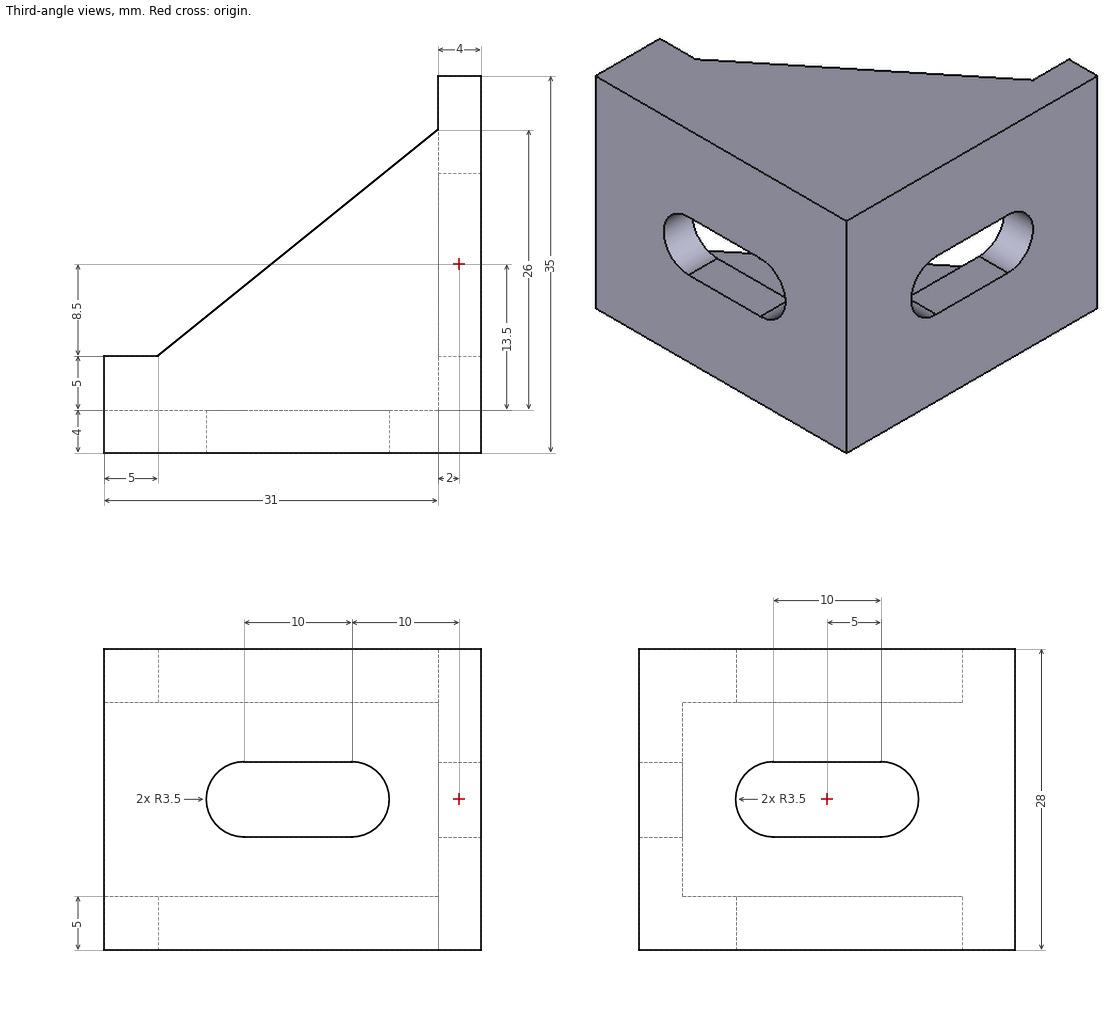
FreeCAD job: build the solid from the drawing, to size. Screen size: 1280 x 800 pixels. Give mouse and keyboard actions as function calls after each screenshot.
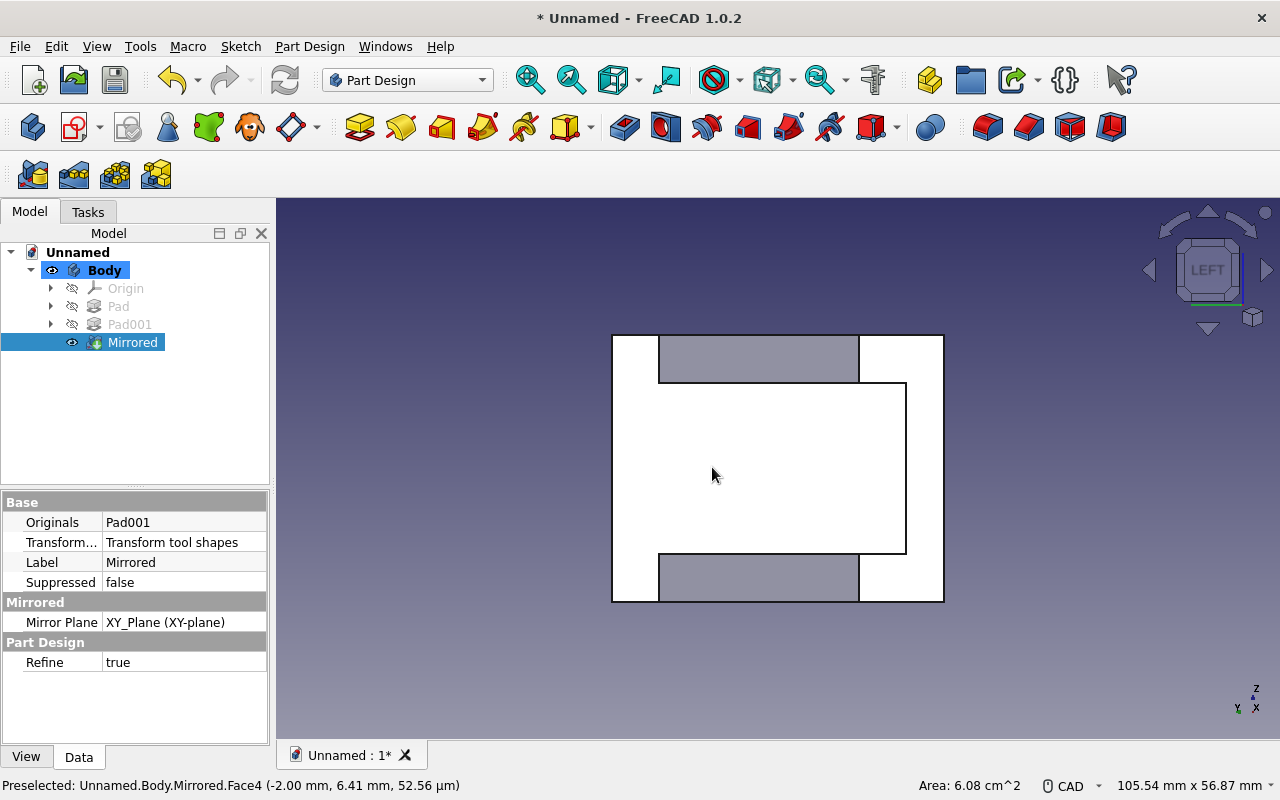
click(74, 128)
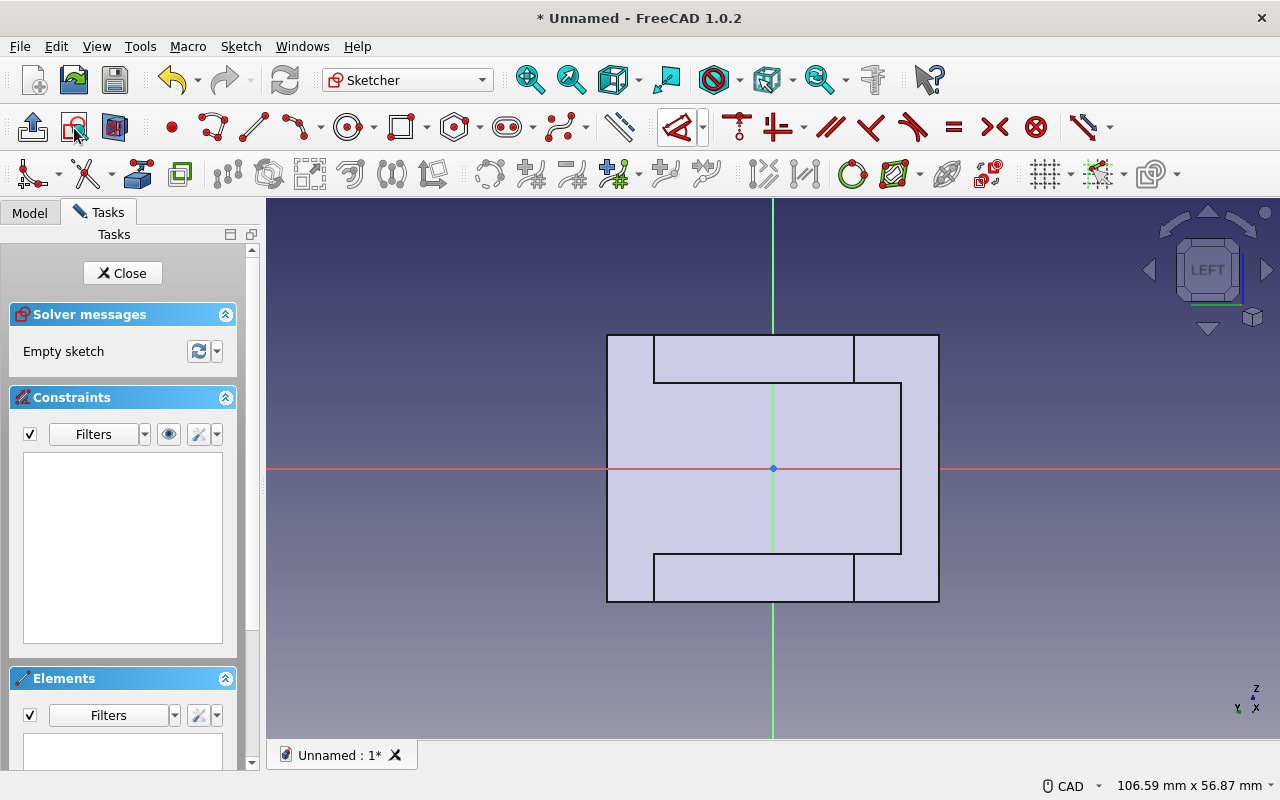
scroll(803, 468, up, 6)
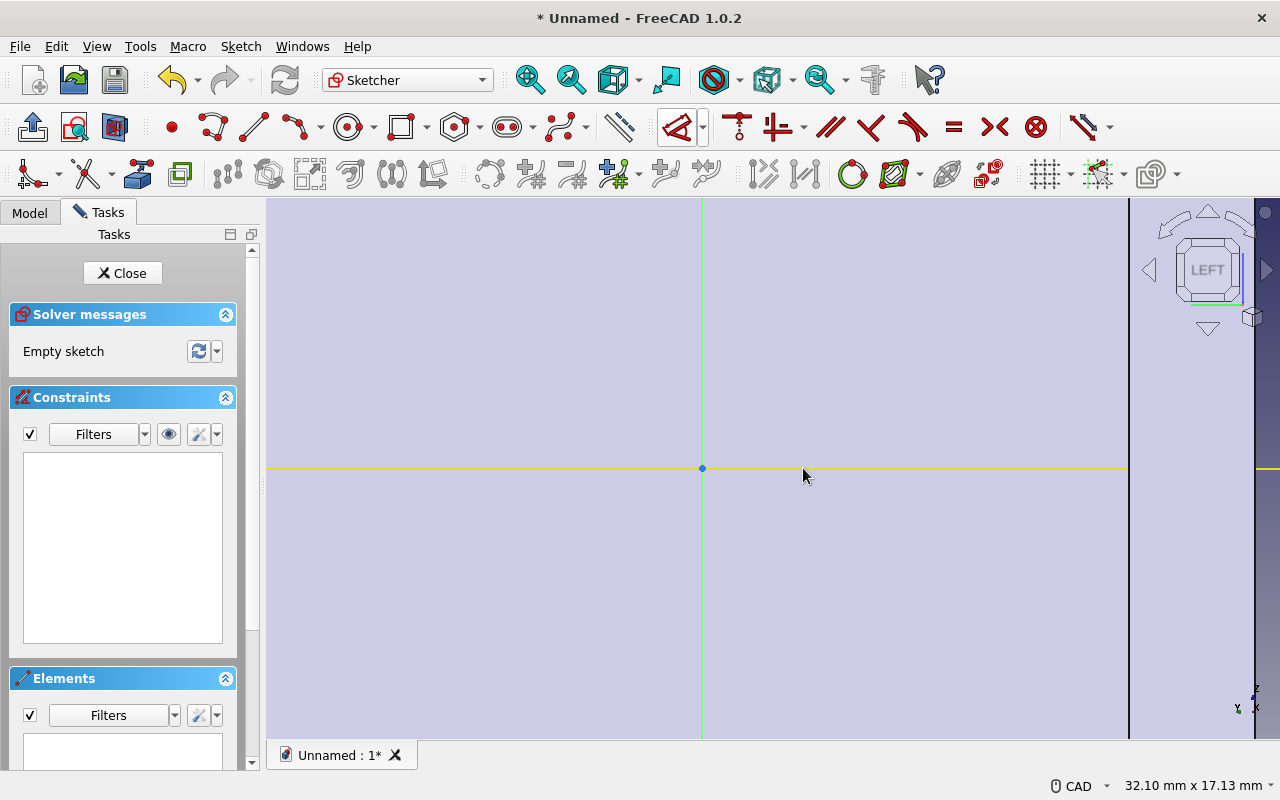
click(506, 128)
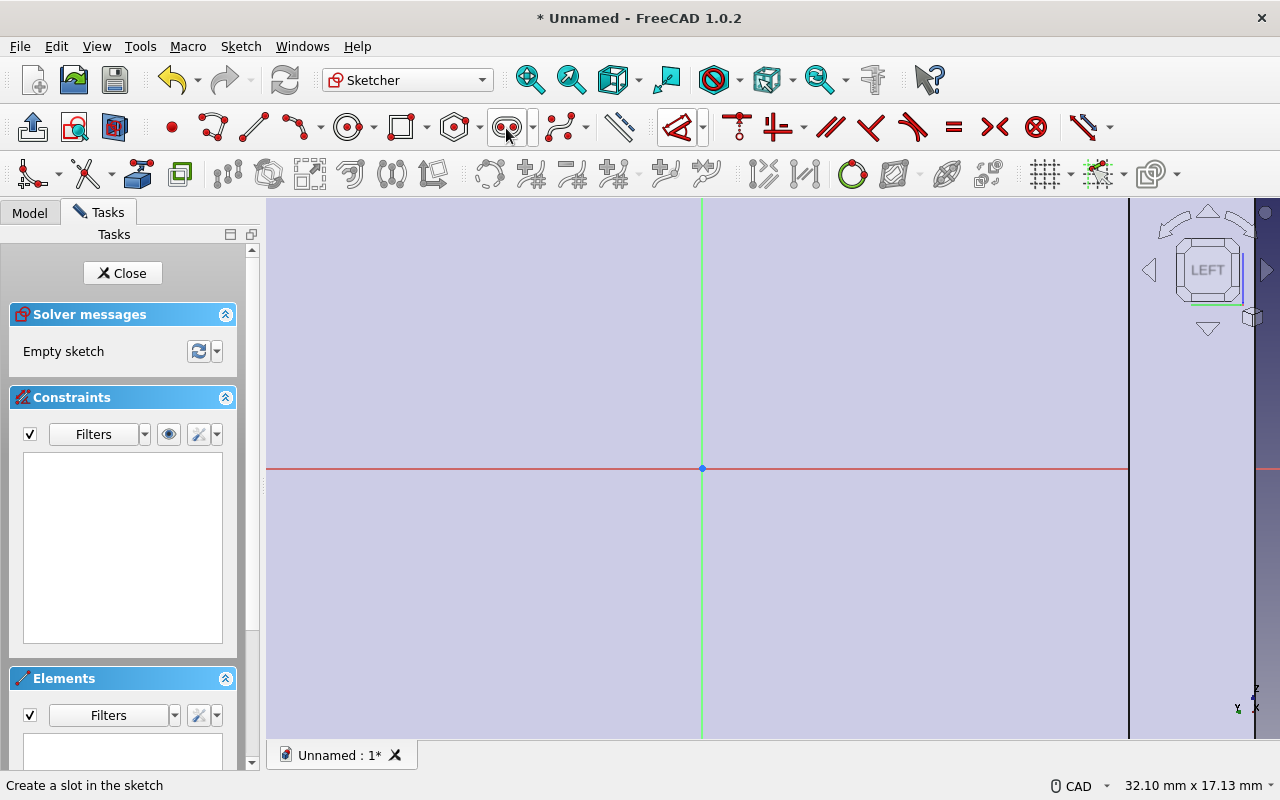
click(544, 468)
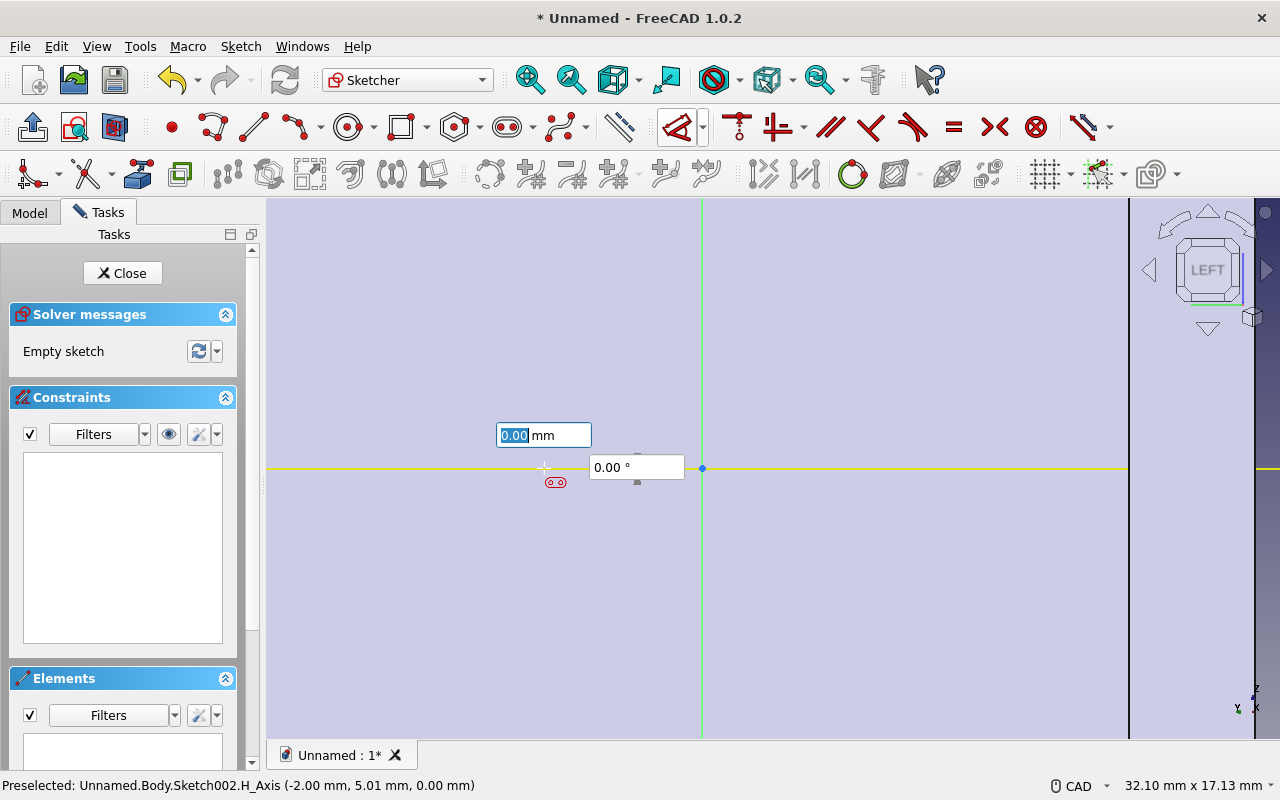
click(860, 460)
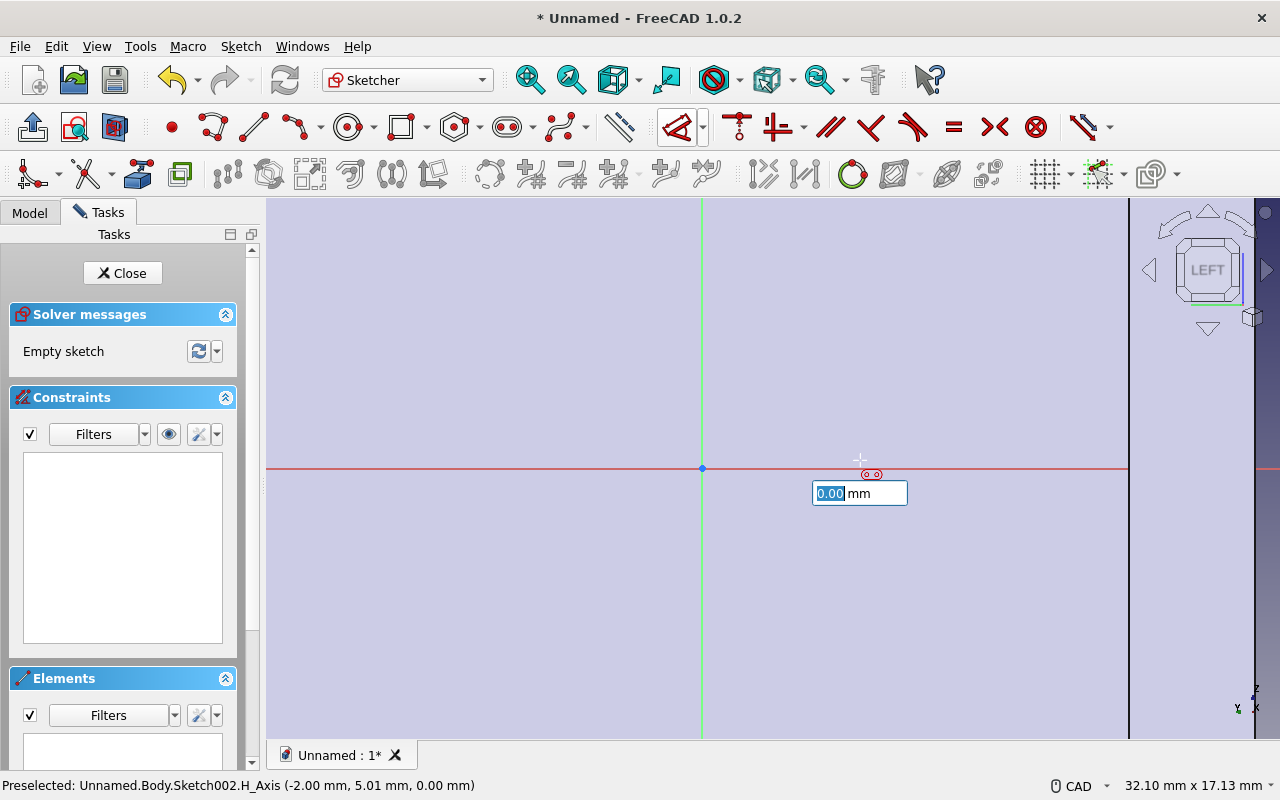
click(655, 579)
key(Escape)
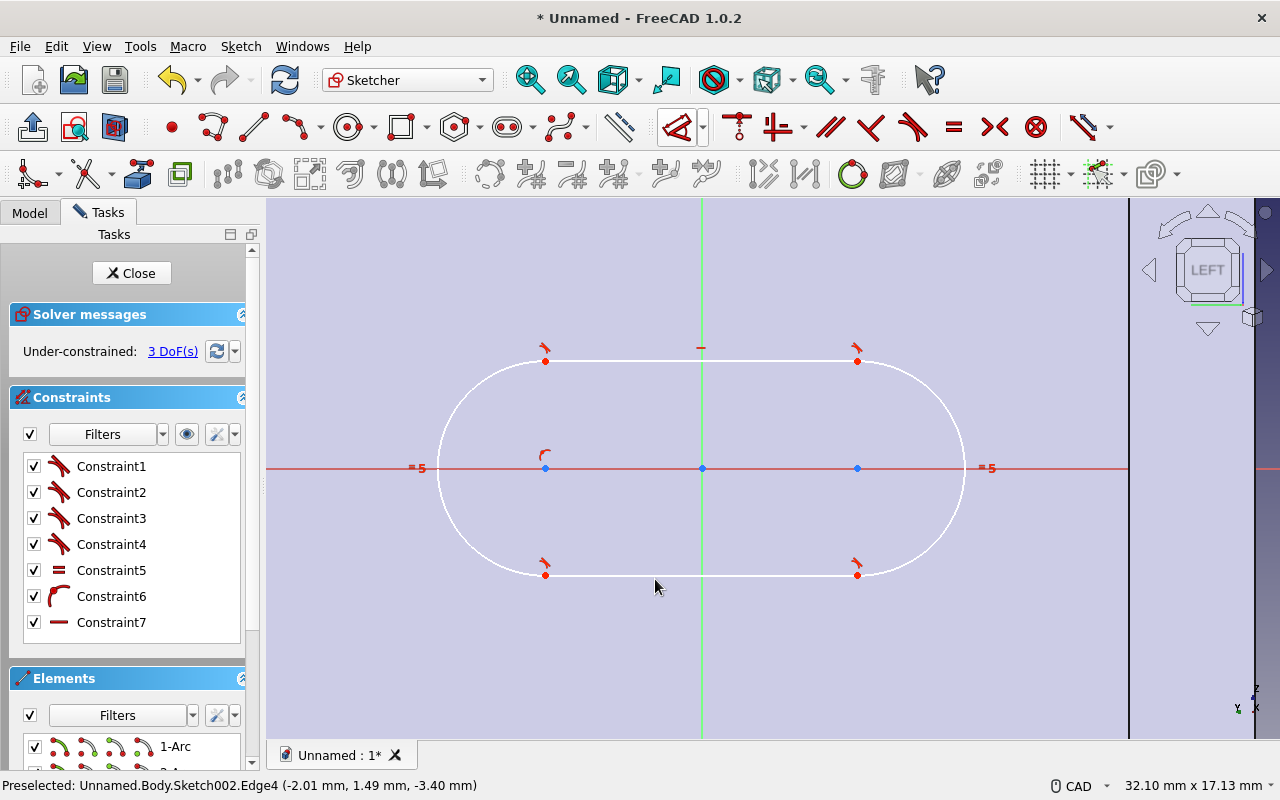
click(458, 405)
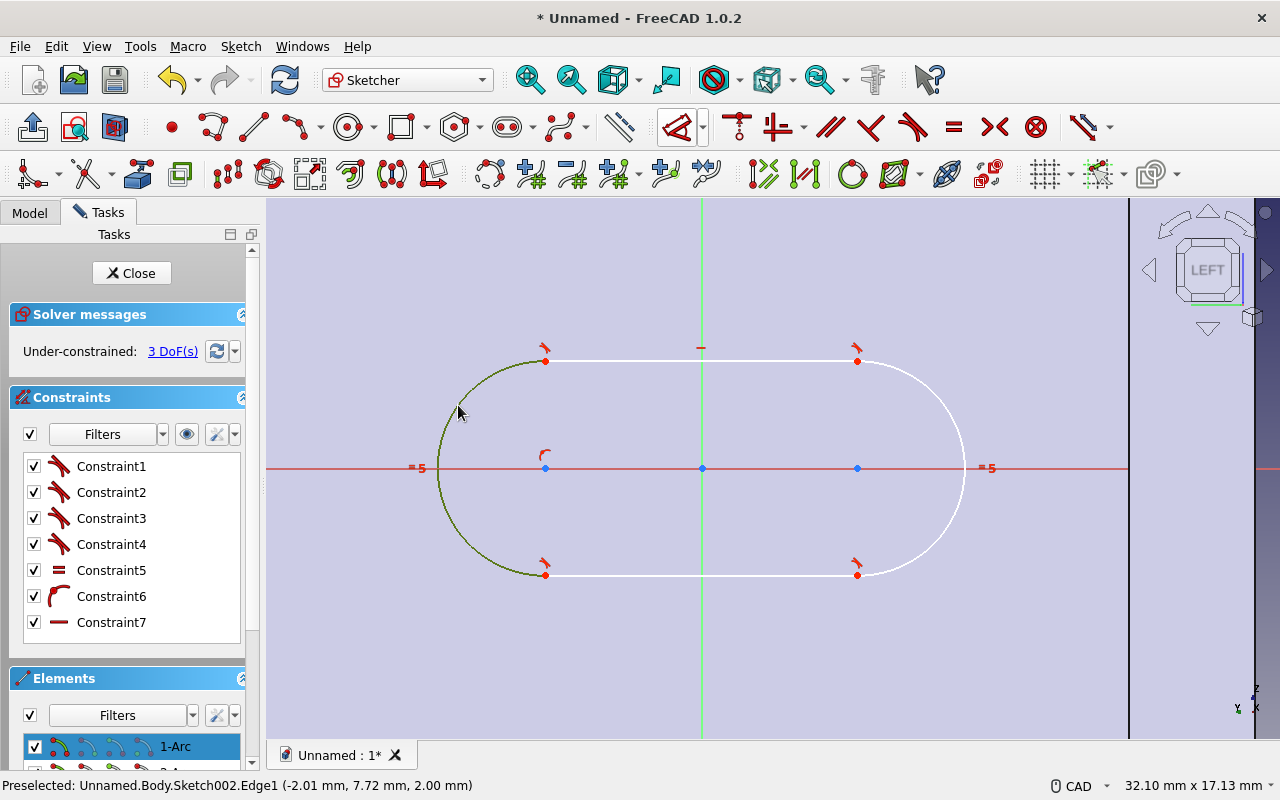
key(k)
key(r)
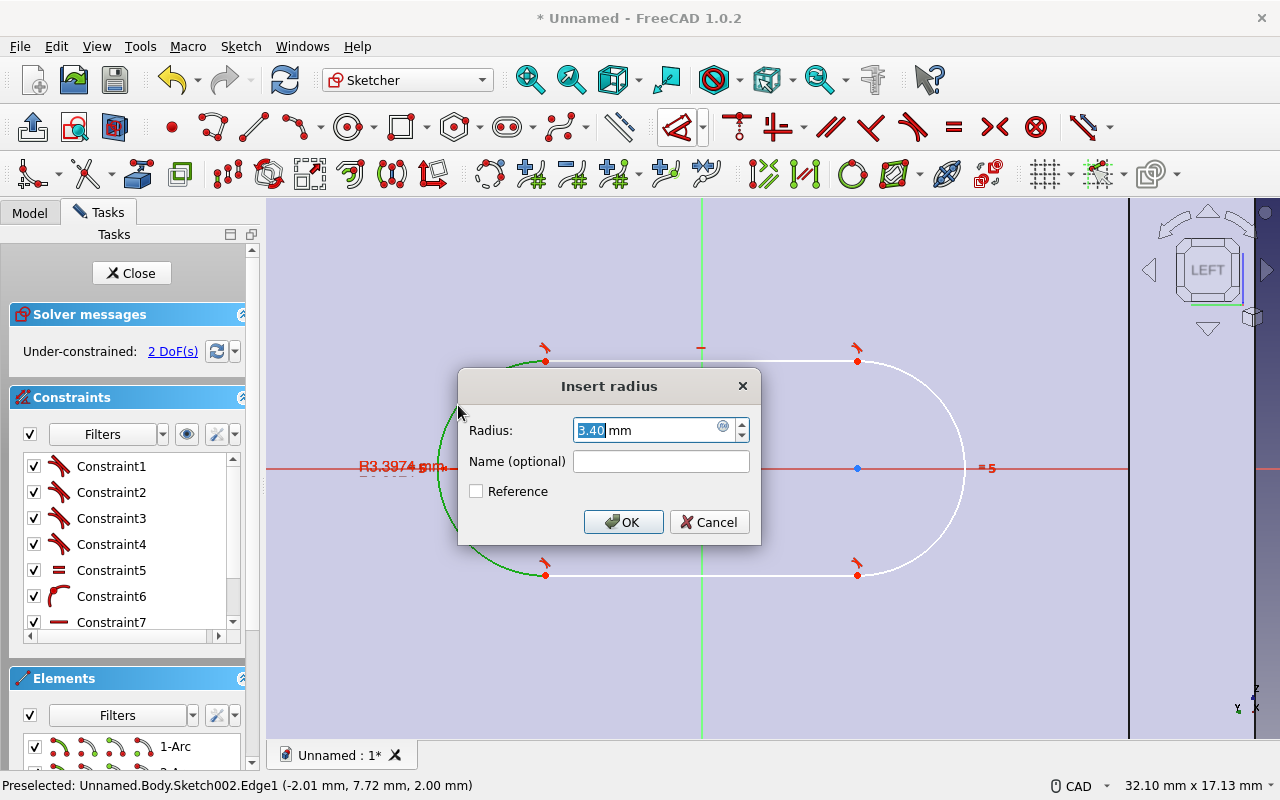
text(3.5)
key(Return)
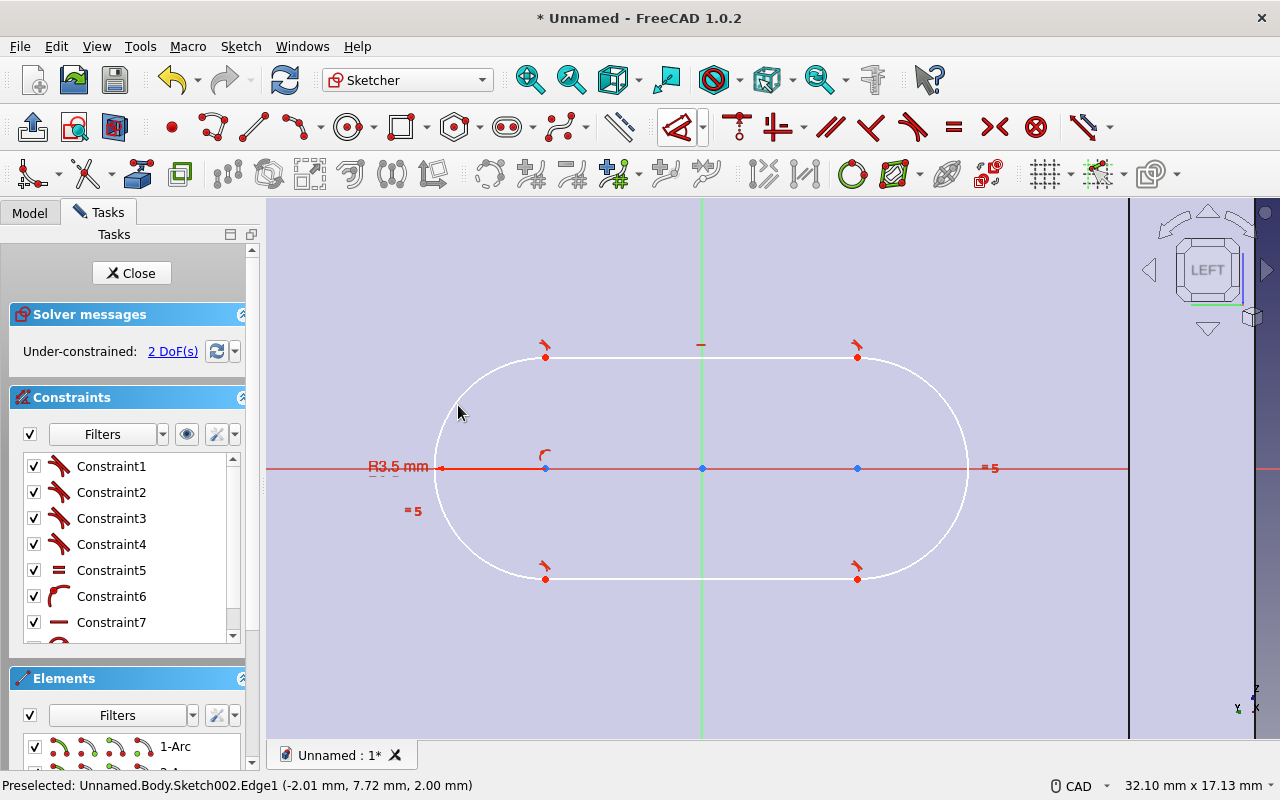
click(639, 358)